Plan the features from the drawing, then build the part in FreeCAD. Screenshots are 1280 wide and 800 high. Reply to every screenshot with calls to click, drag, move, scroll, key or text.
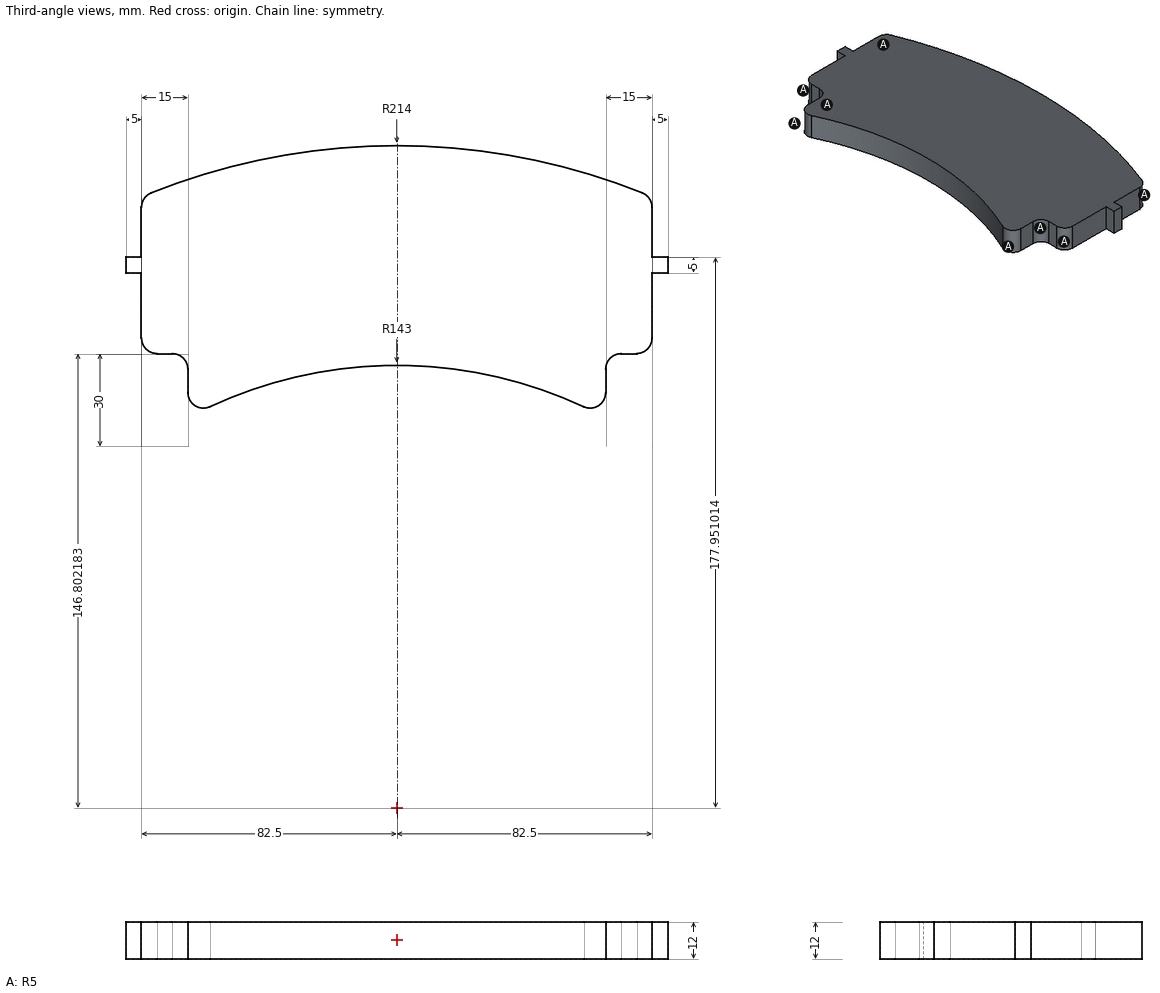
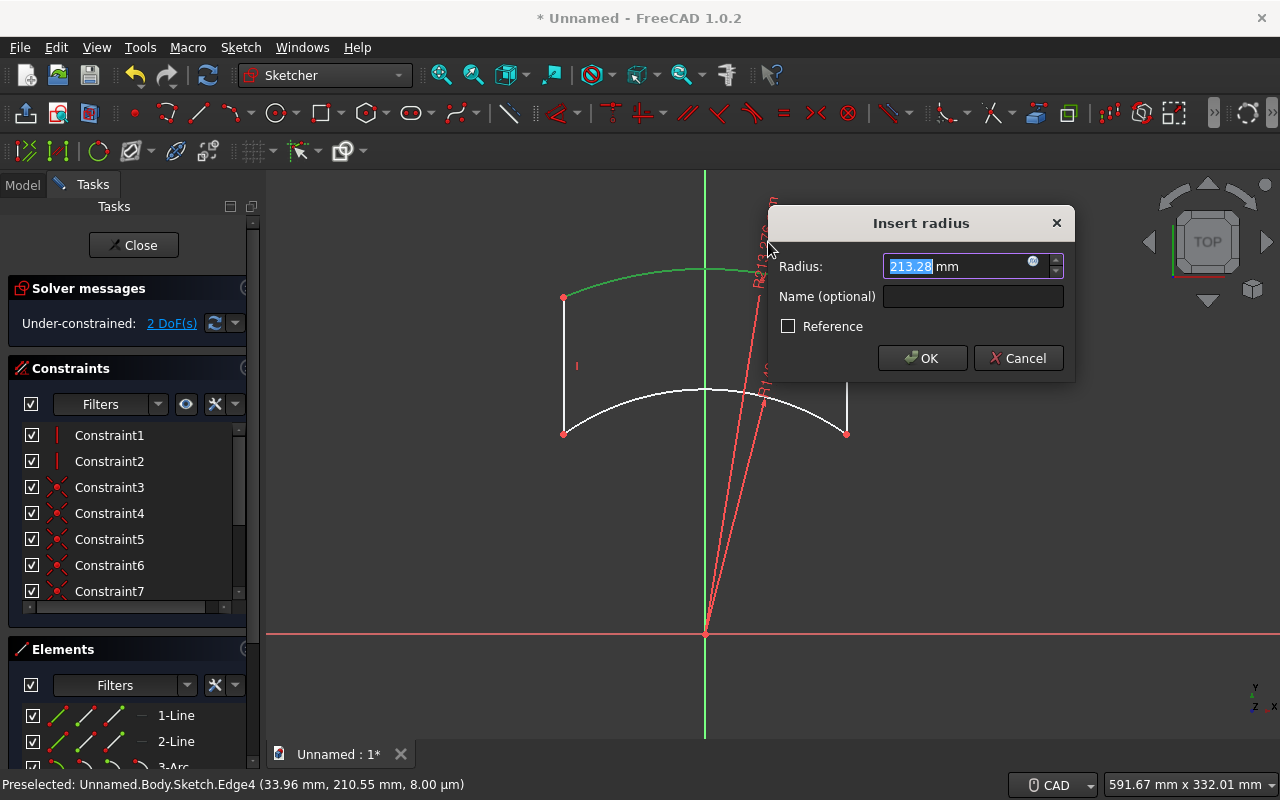
text(214)
key(Return)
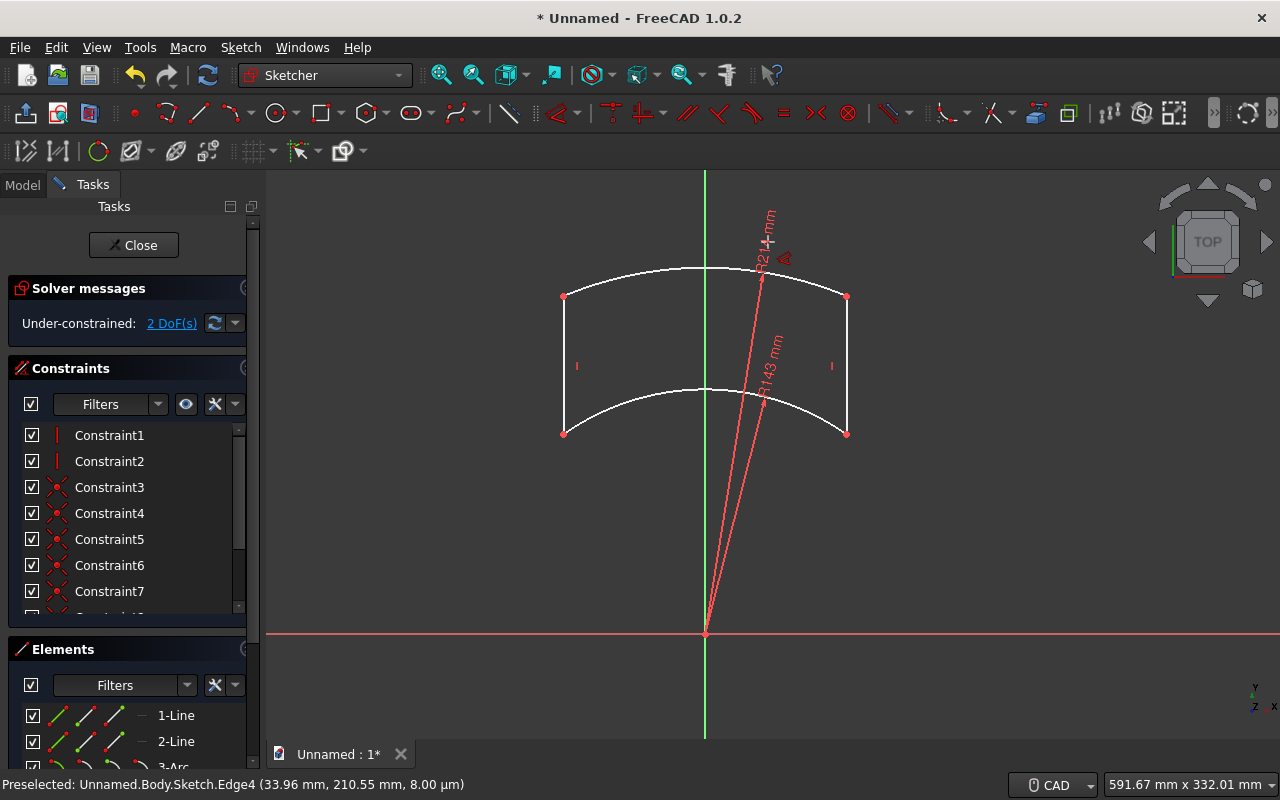
click(564, 296)
click(634, 668)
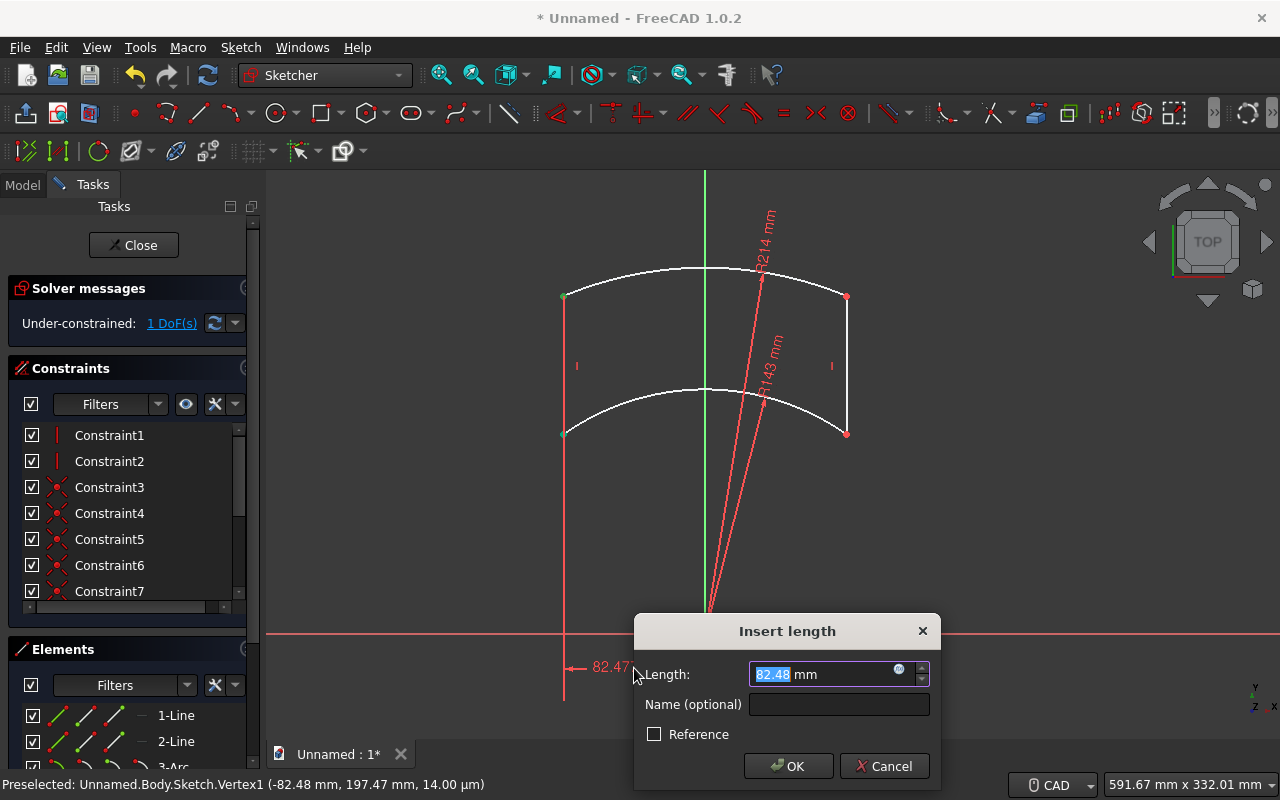
text(82.5)
key(Return)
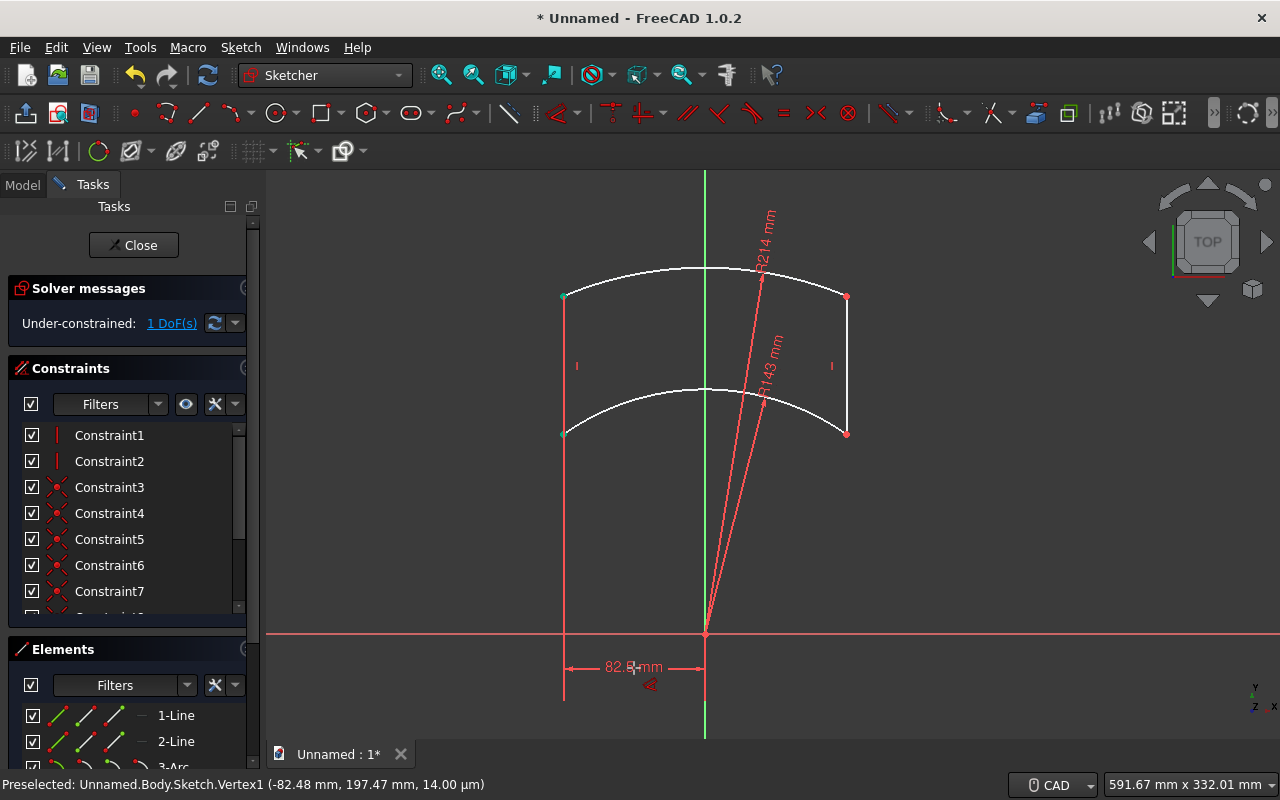
click(847, 435)
click(776, 668)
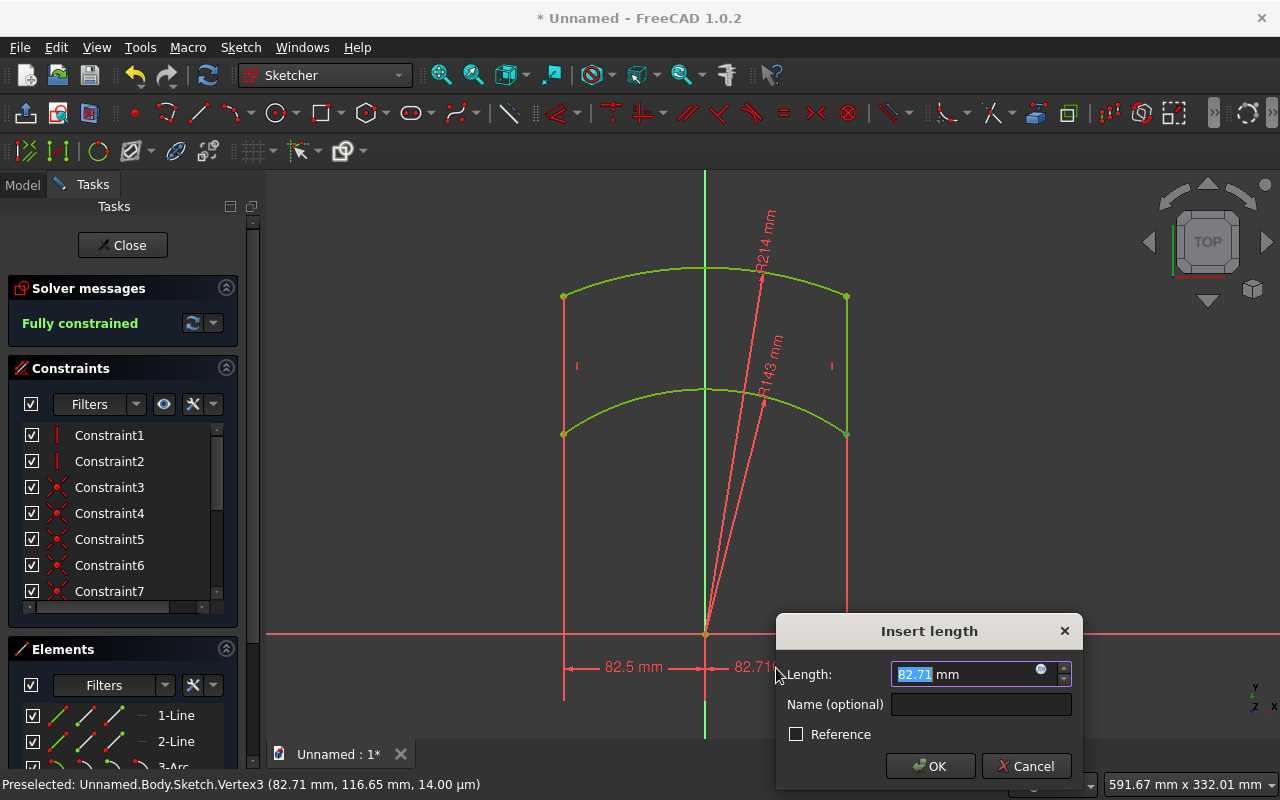
text(82.5)
key(Return)
key(Escape)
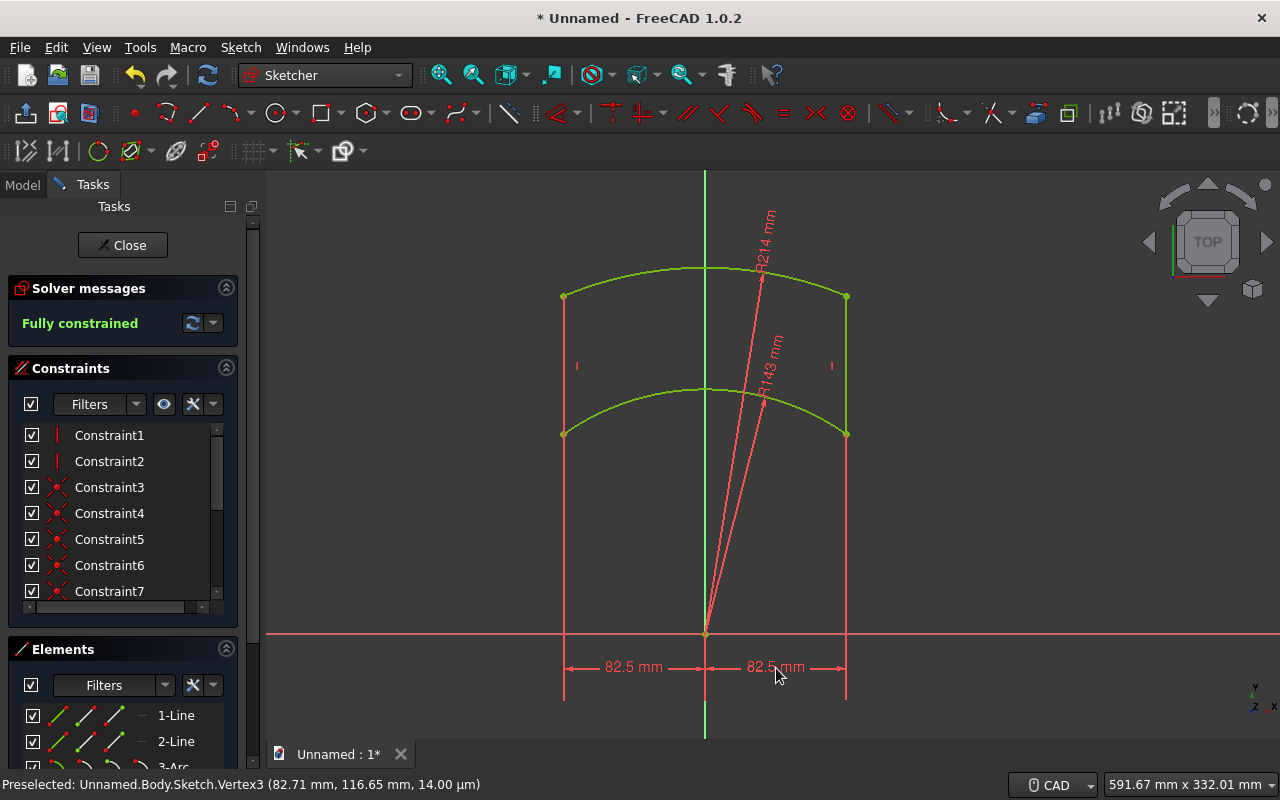
click(123, 245)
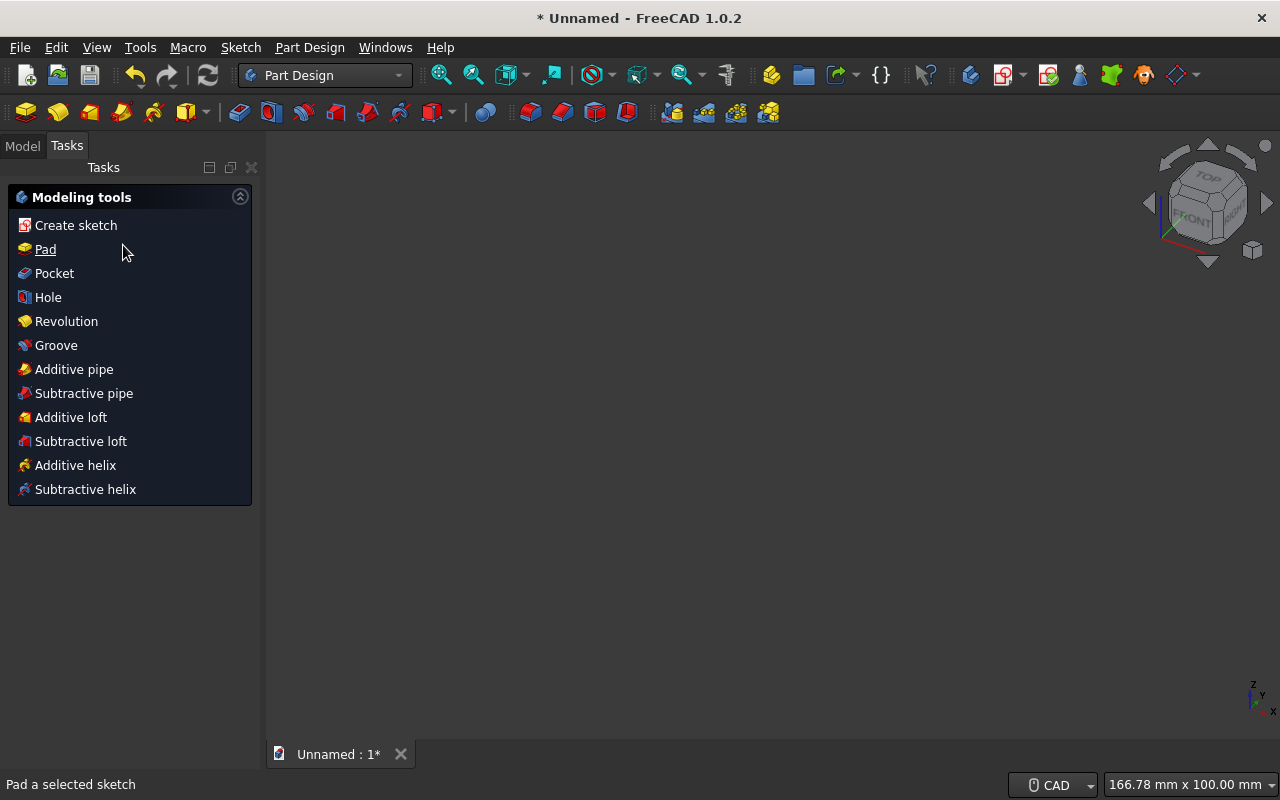
click(26, 112)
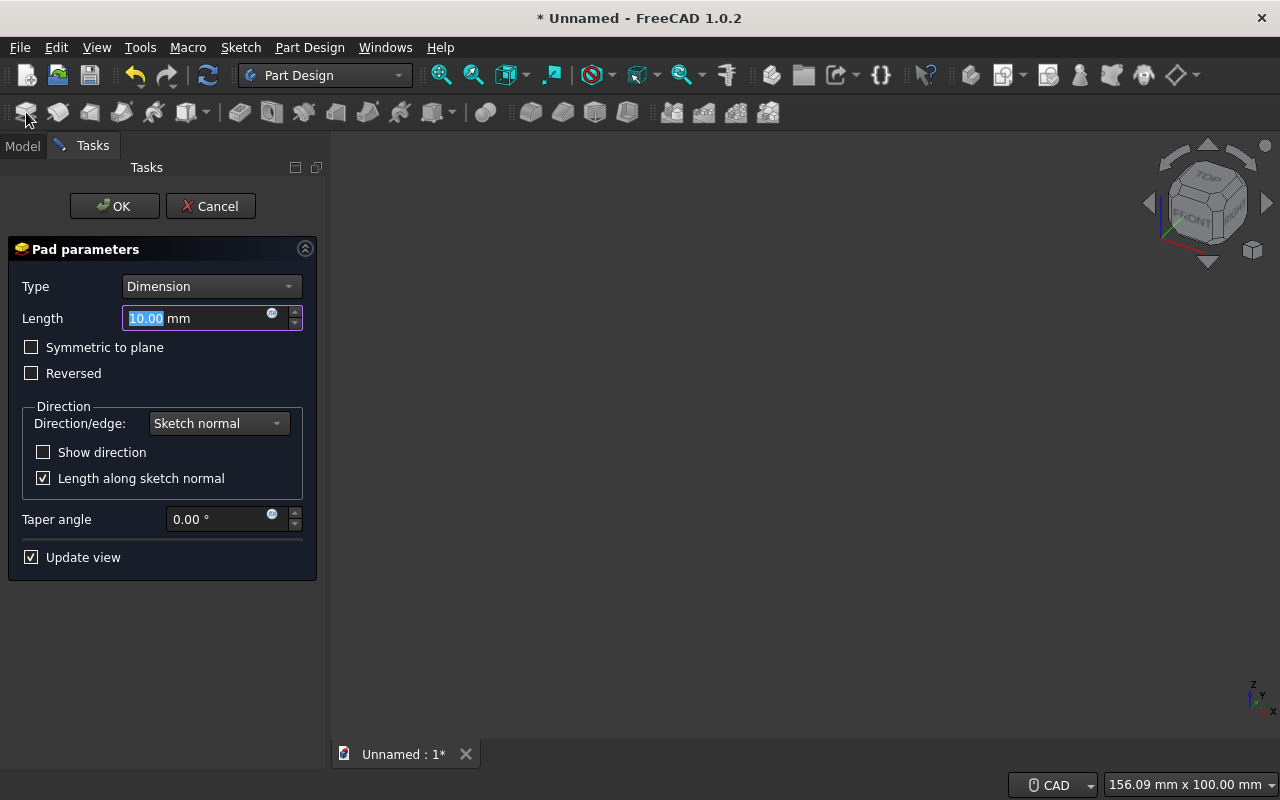
text(12)
key(Tab)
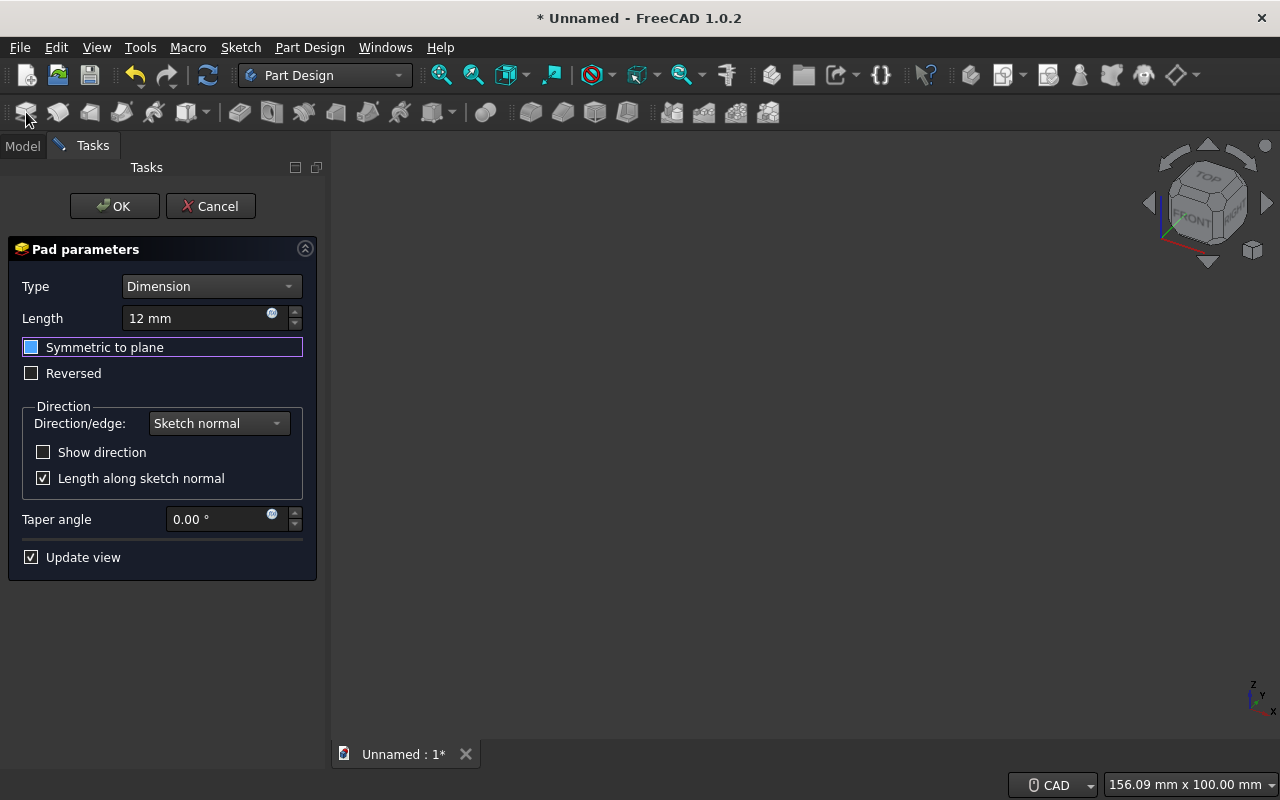
click(30, 347)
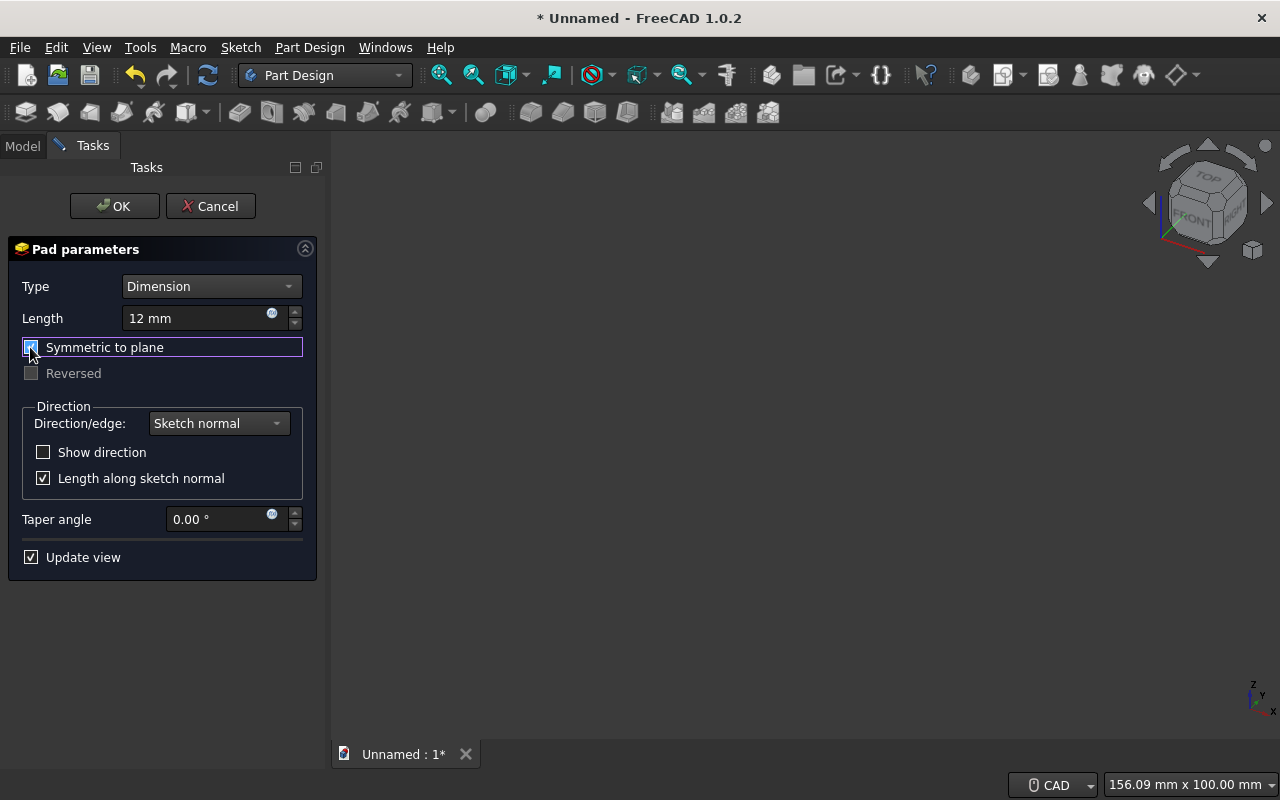
click(115, 206)